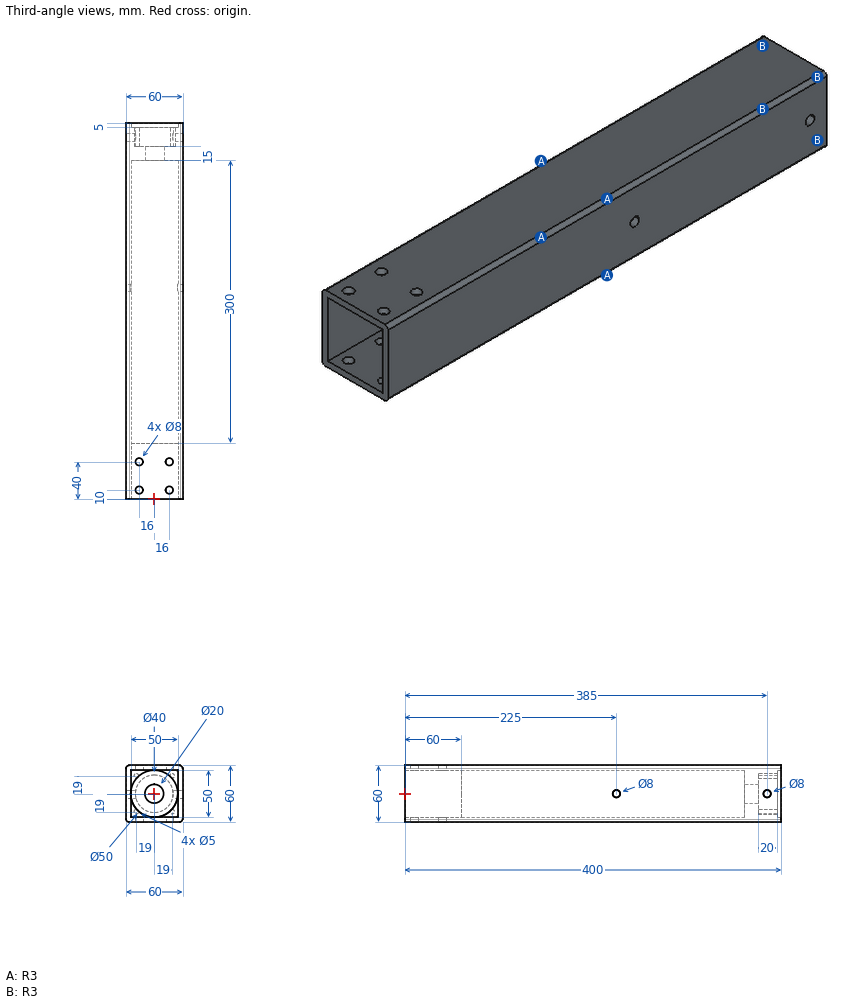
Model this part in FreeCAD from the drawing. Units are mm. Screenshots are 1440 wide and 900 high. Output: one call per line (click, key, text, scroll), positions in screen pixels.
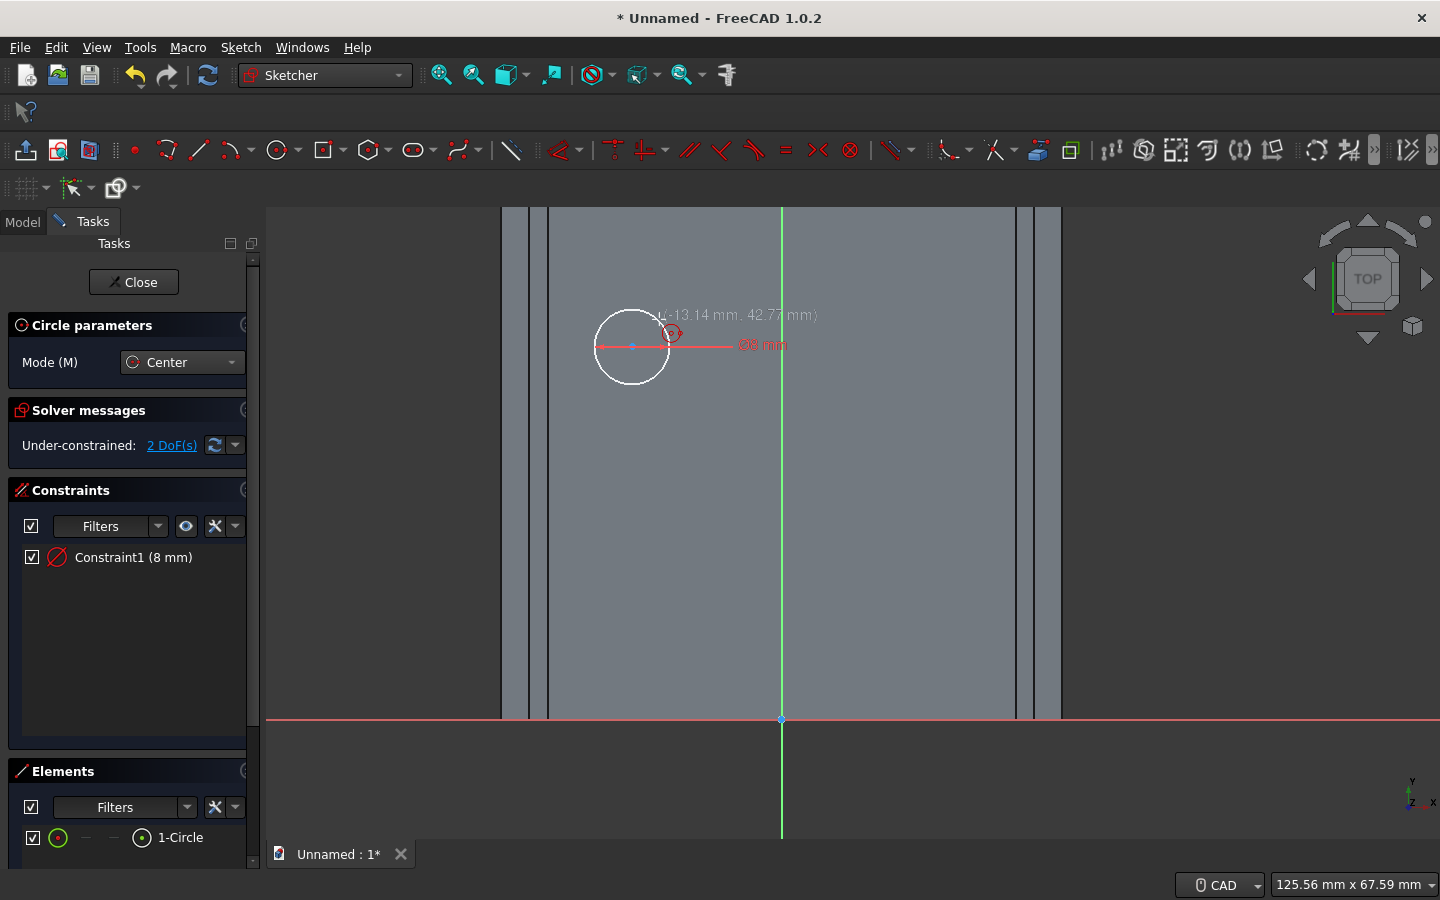
click(632, 626)
move(659, 600)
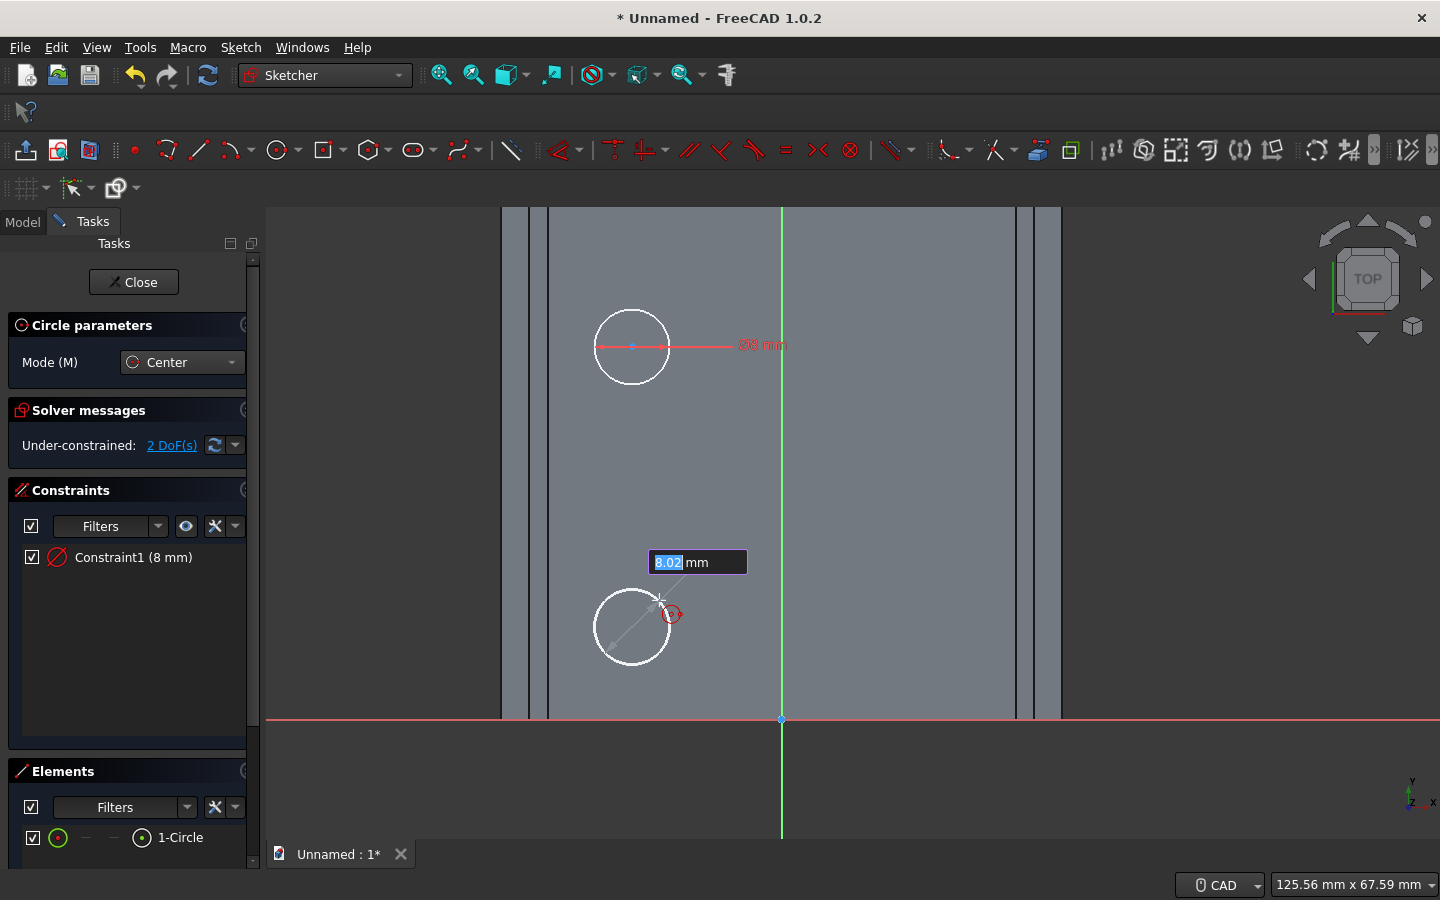
text(8)
key(Return)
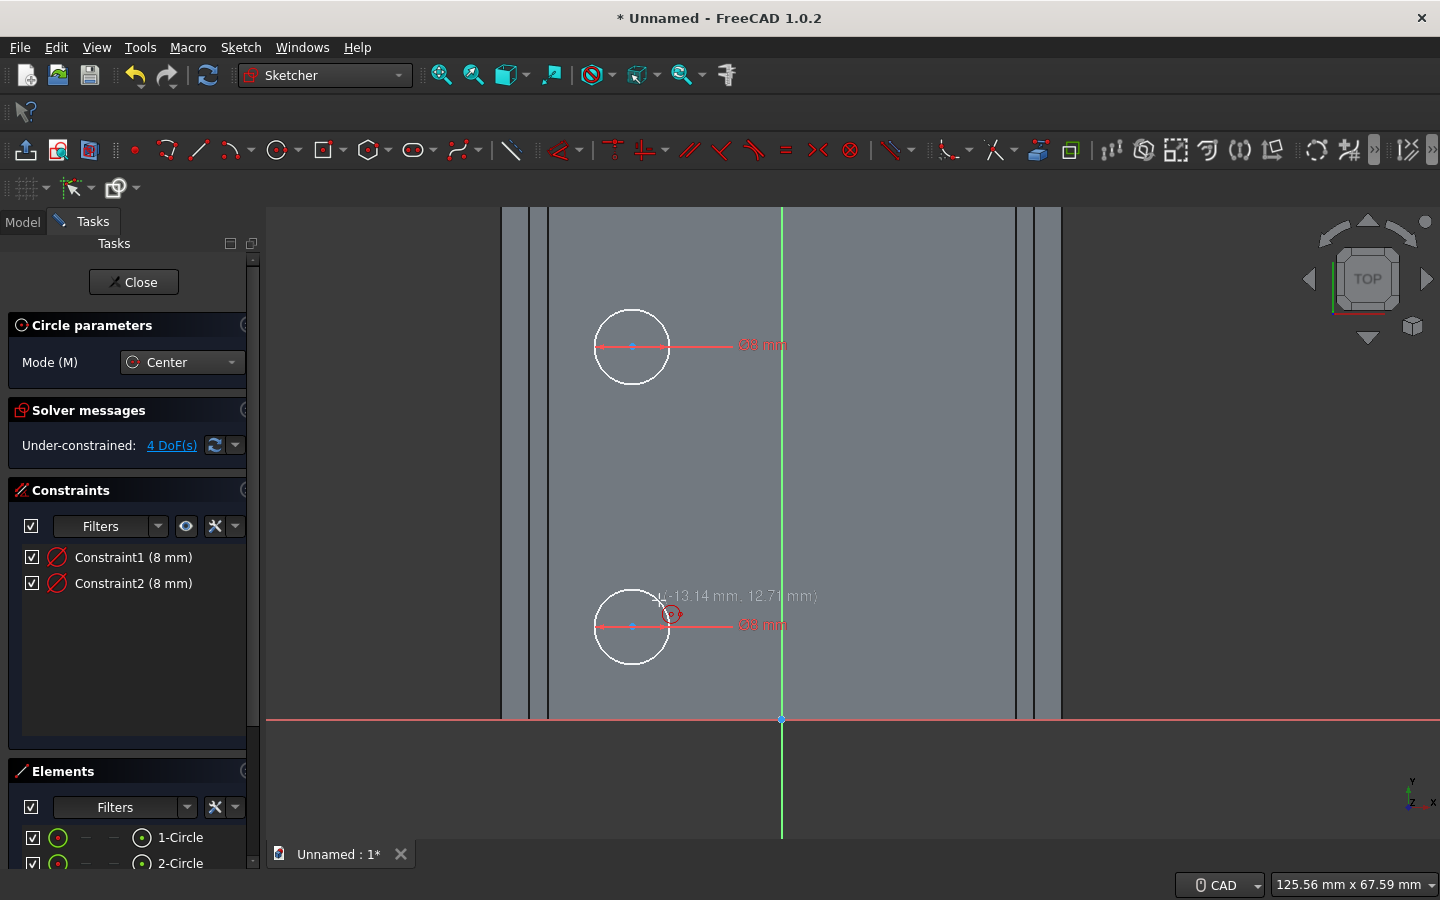
click(931, 626)
move(958, 600)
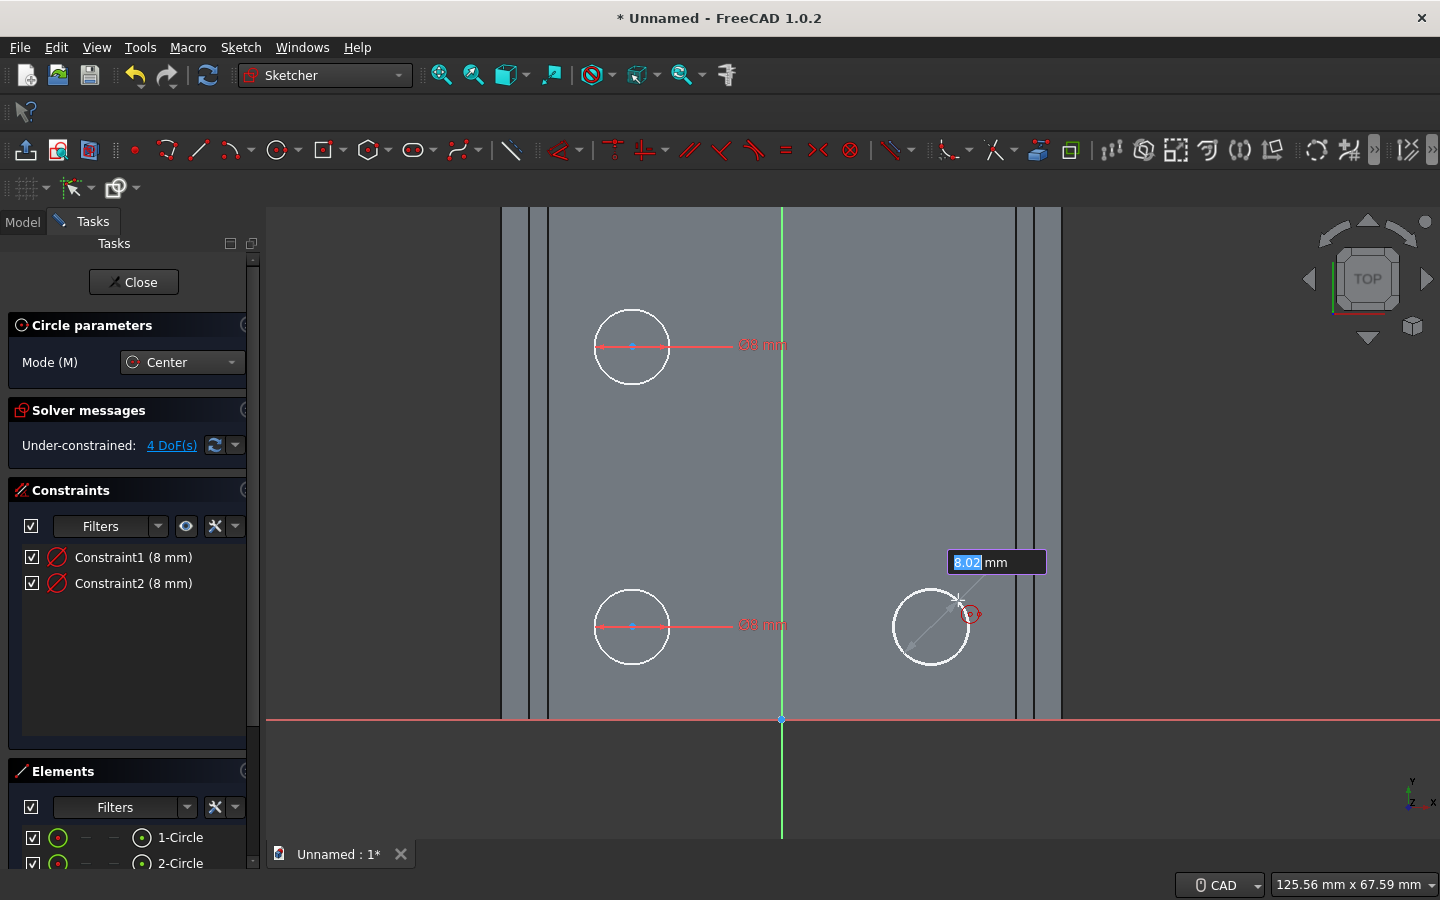
text(8)
key(Return)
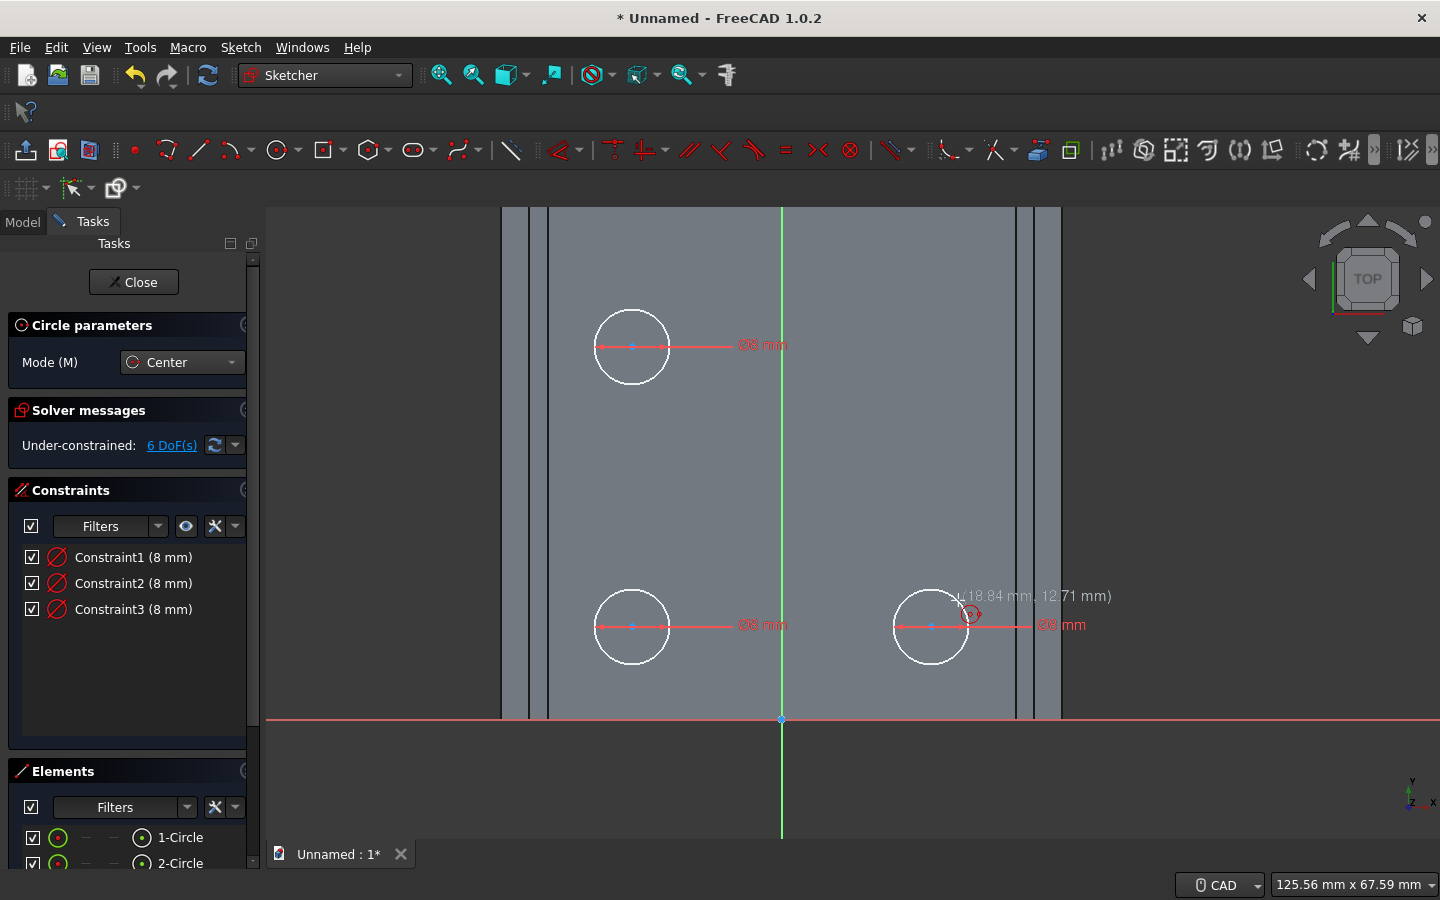
click(931, 346)
move(958, 319)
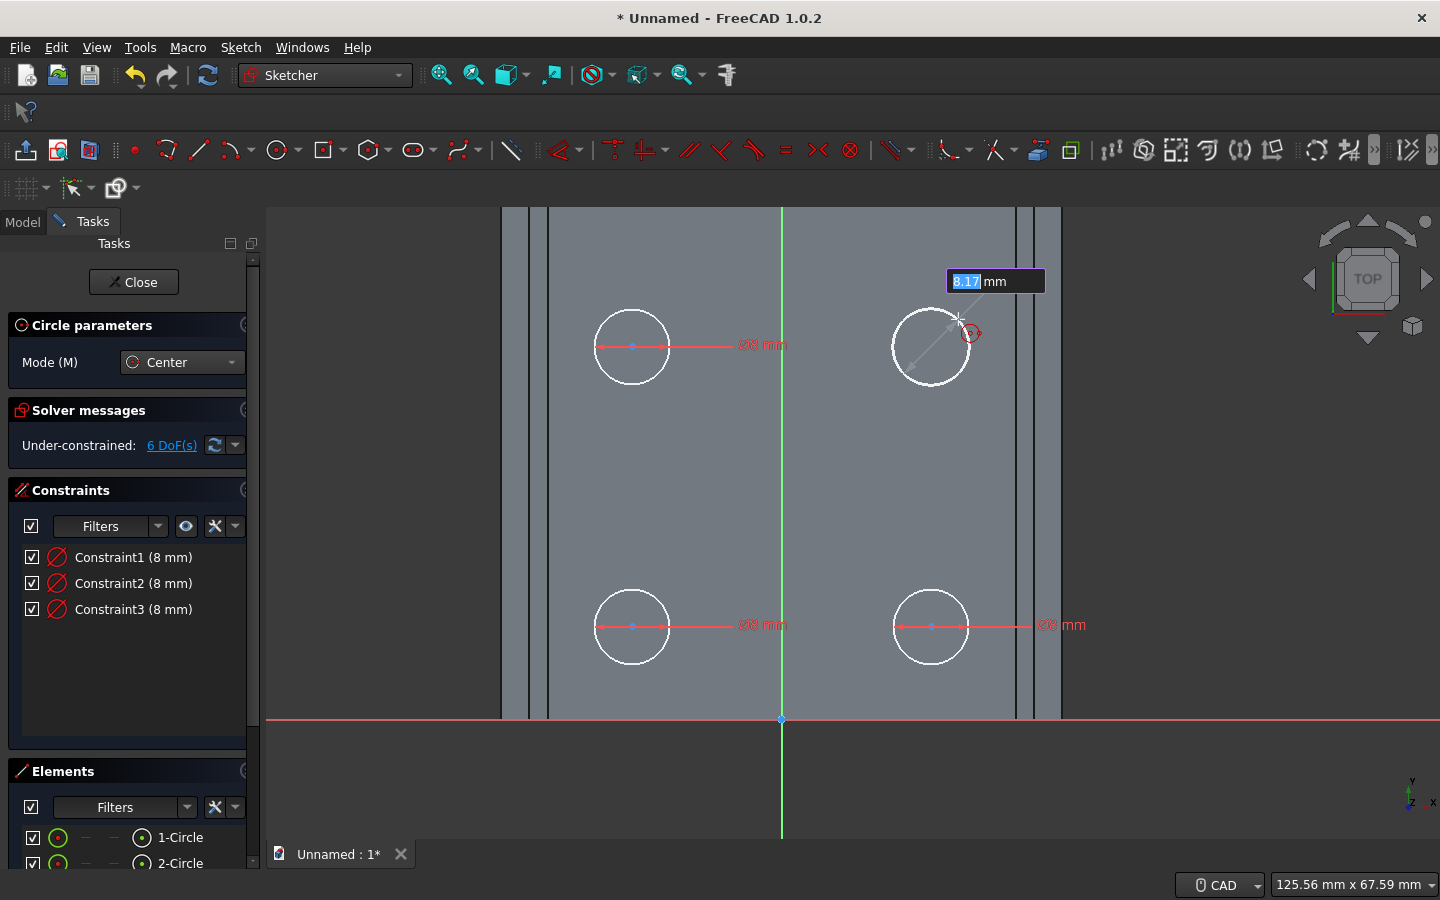
text(8)
key(Return)
key(Escape)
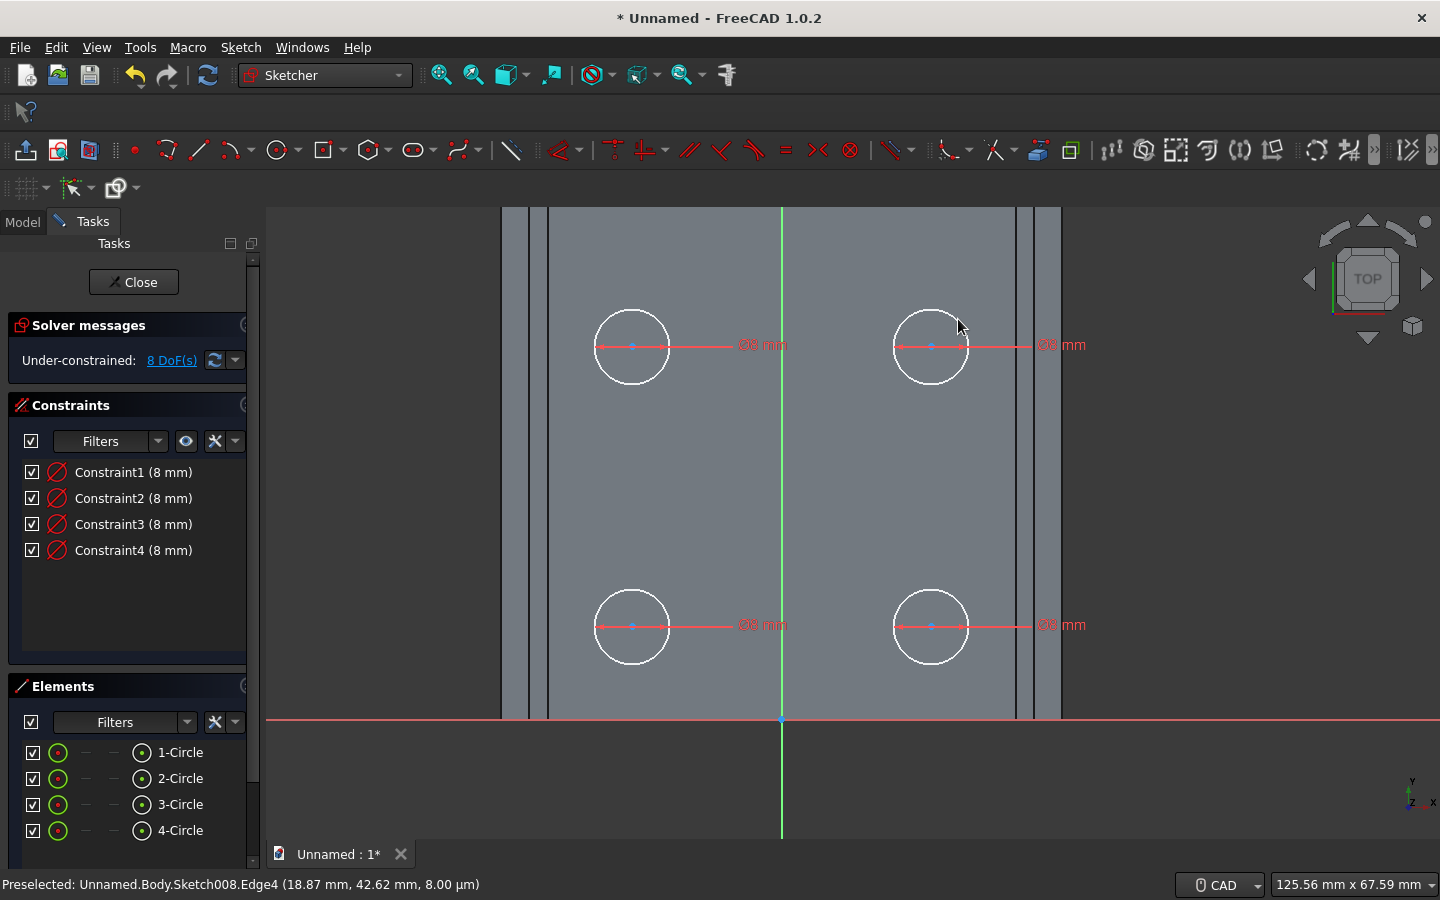
click(632, 347)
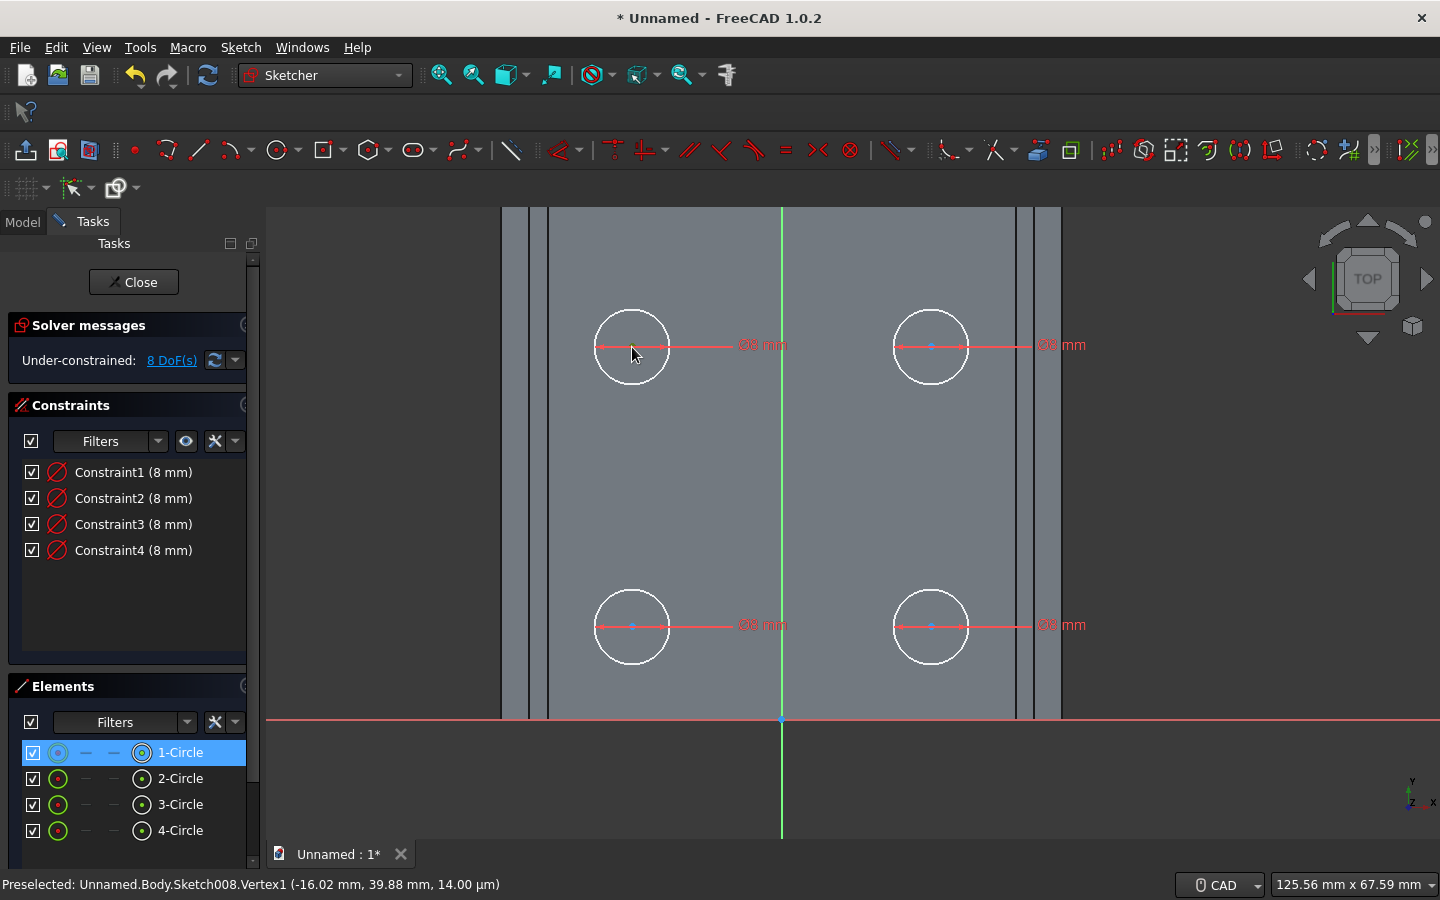
click(632, 627)